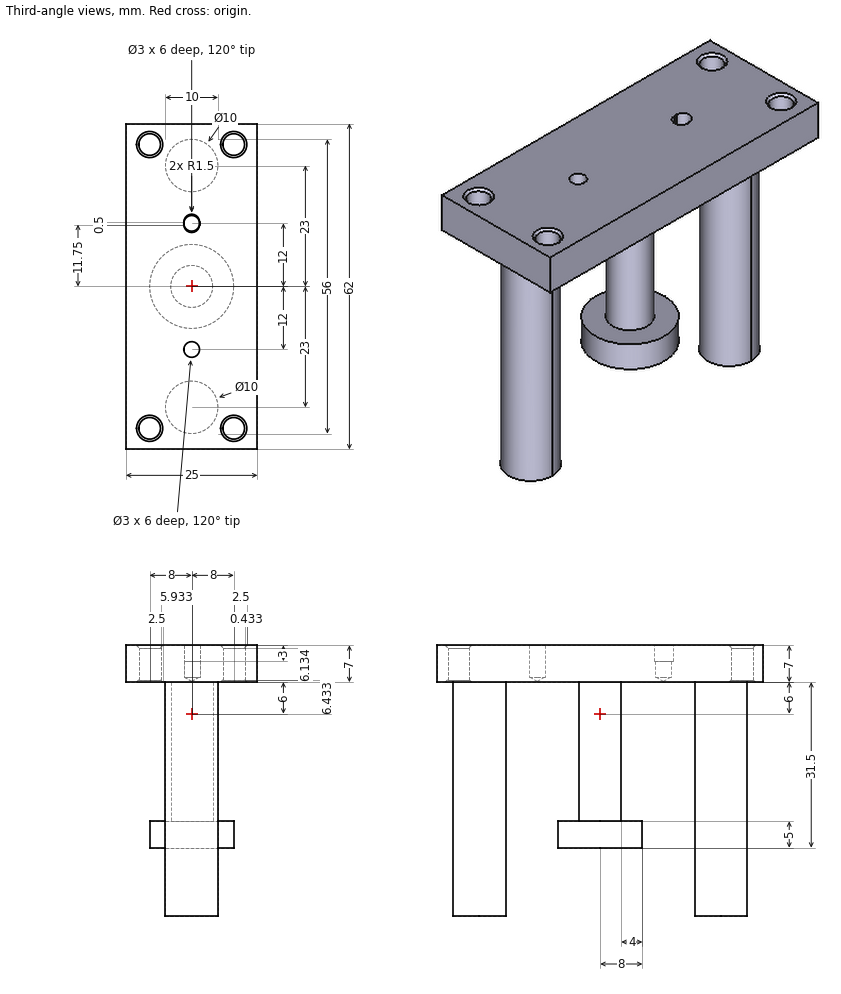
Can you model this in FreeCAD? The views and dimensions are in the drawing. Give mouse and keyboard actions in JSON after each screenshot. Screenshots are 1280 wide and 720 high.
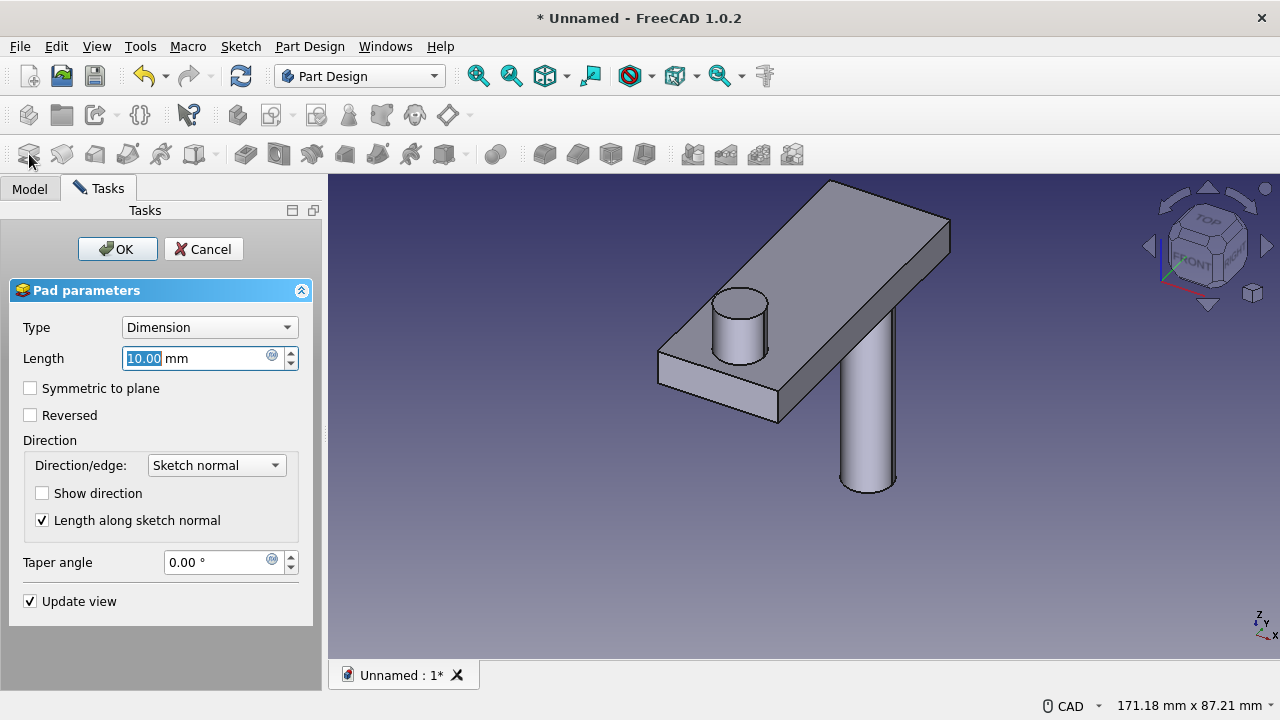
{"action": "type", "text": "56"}
{"action": "key", "text": "Tab"}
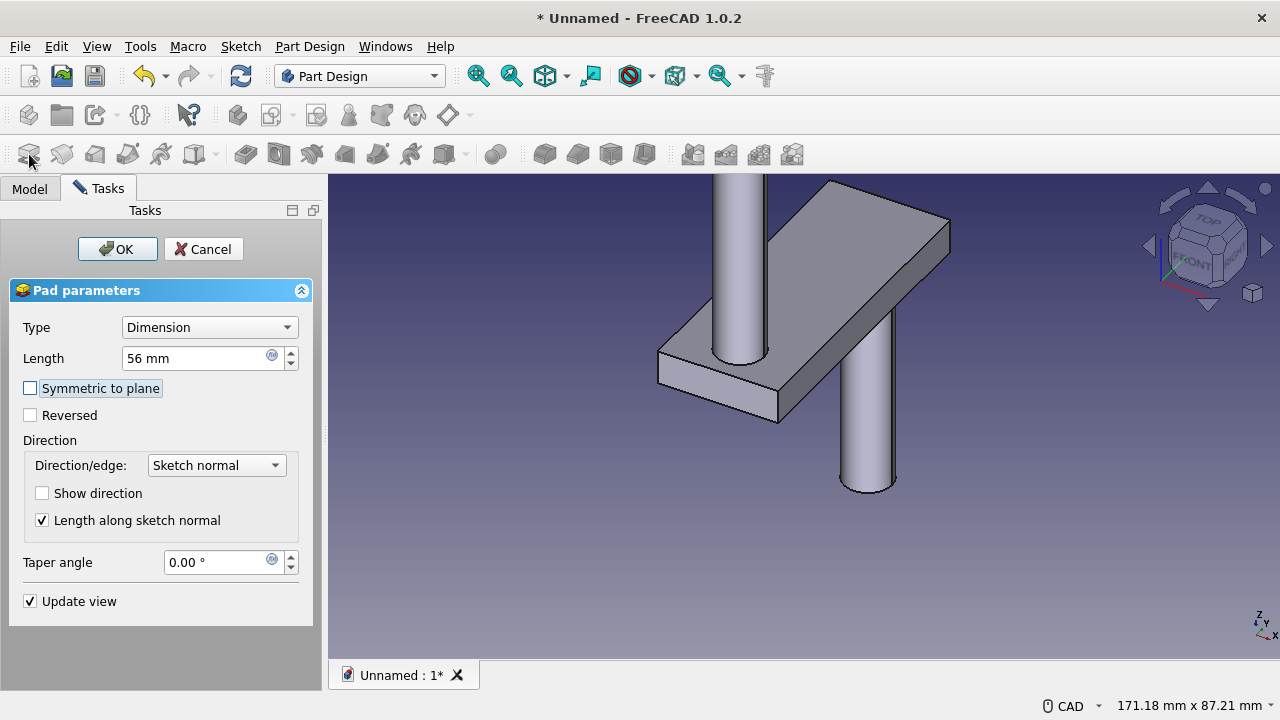
{"action": "left_click", "coordinate": [31, 415]}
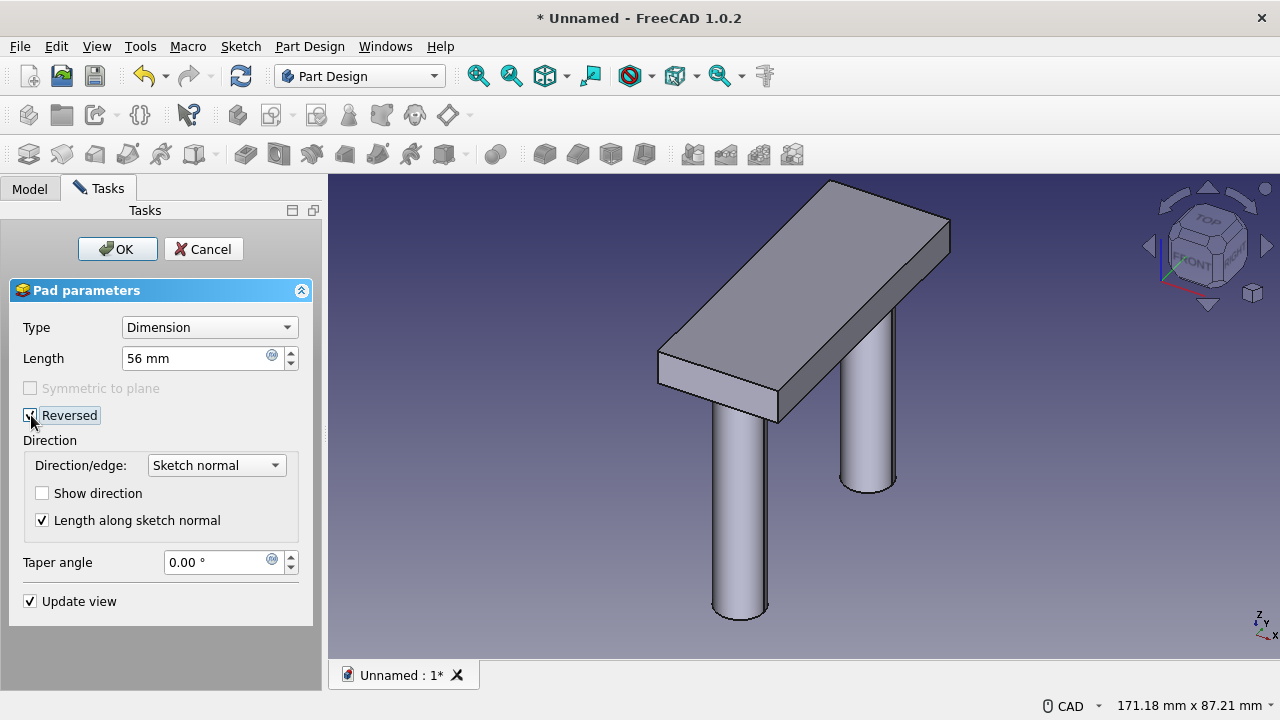
{"action": "left_click", "coordinate": [118, 249]}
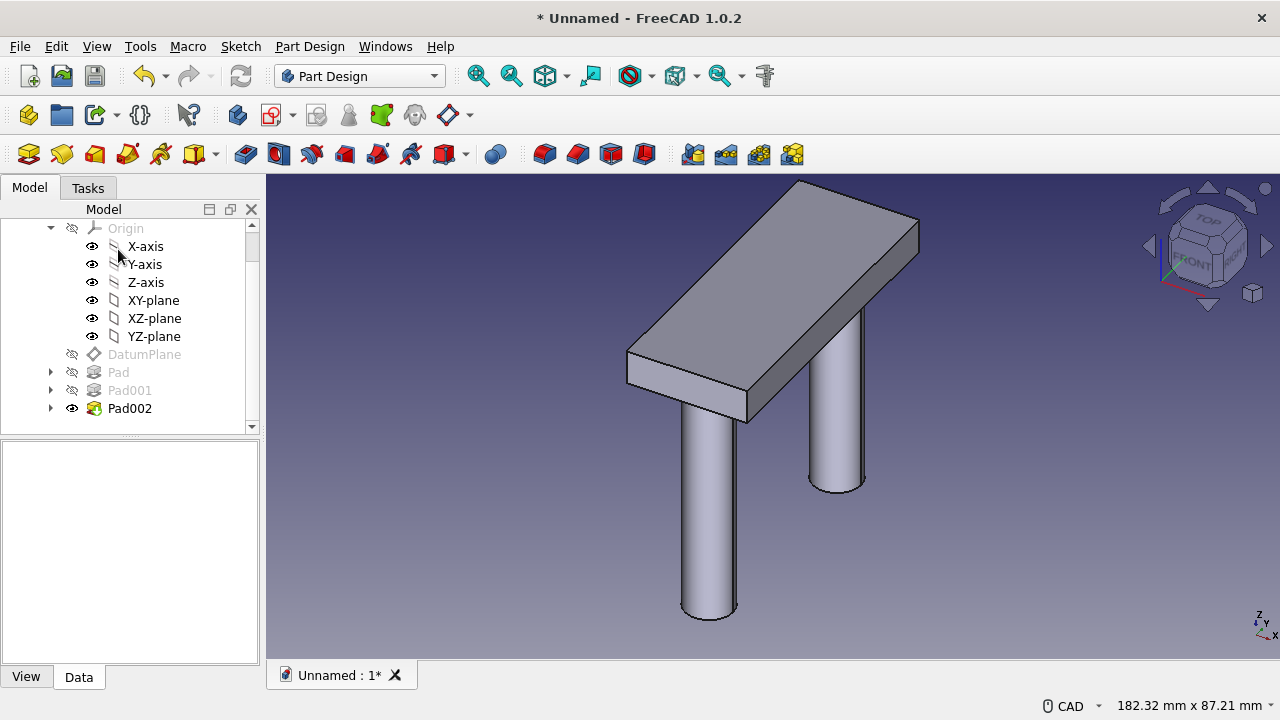
{"action": "left_click", "coordinate": [270, 116]}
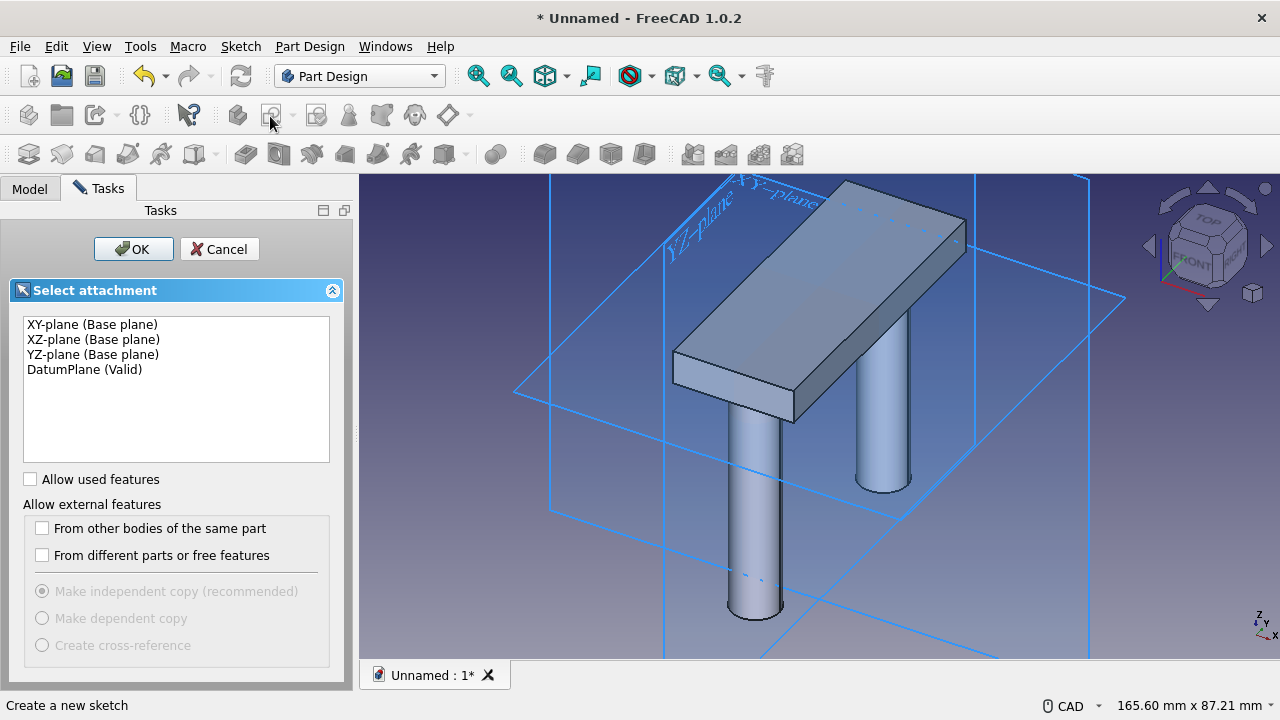
{"action": "left_click", "coordinate": [84, 354]}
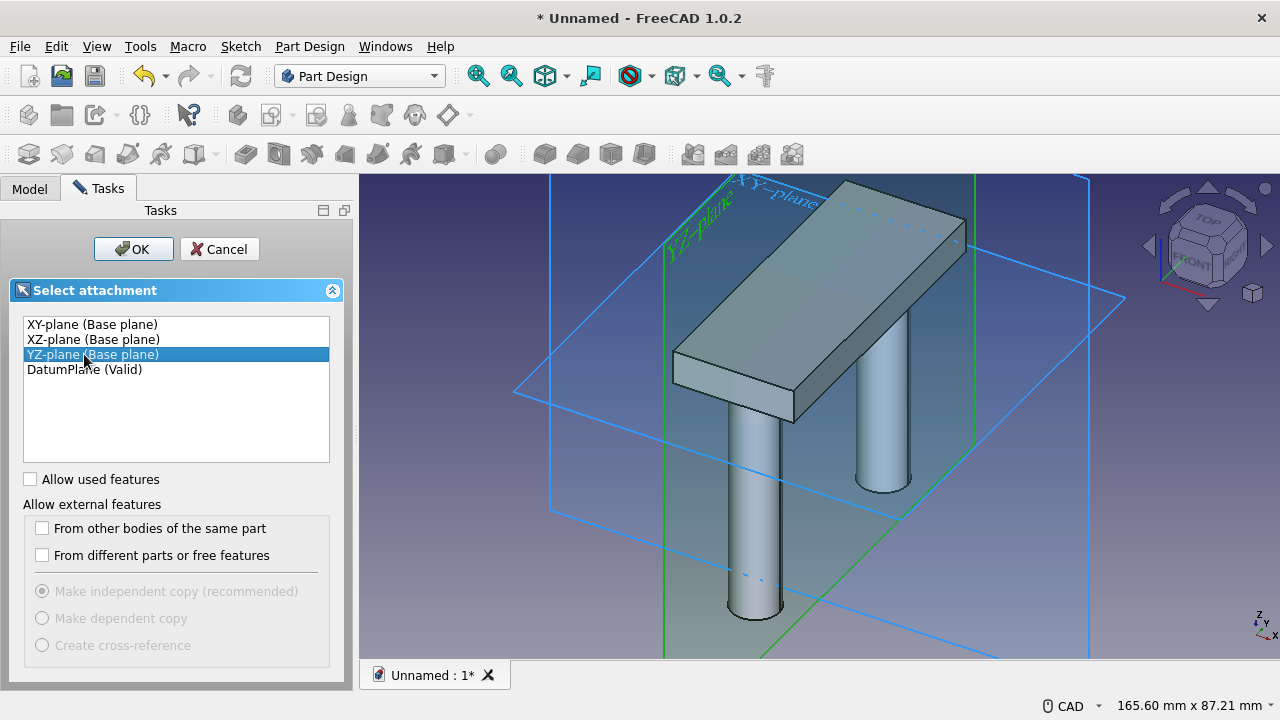
{"action": "left_click", "coordinate": [134, 249]}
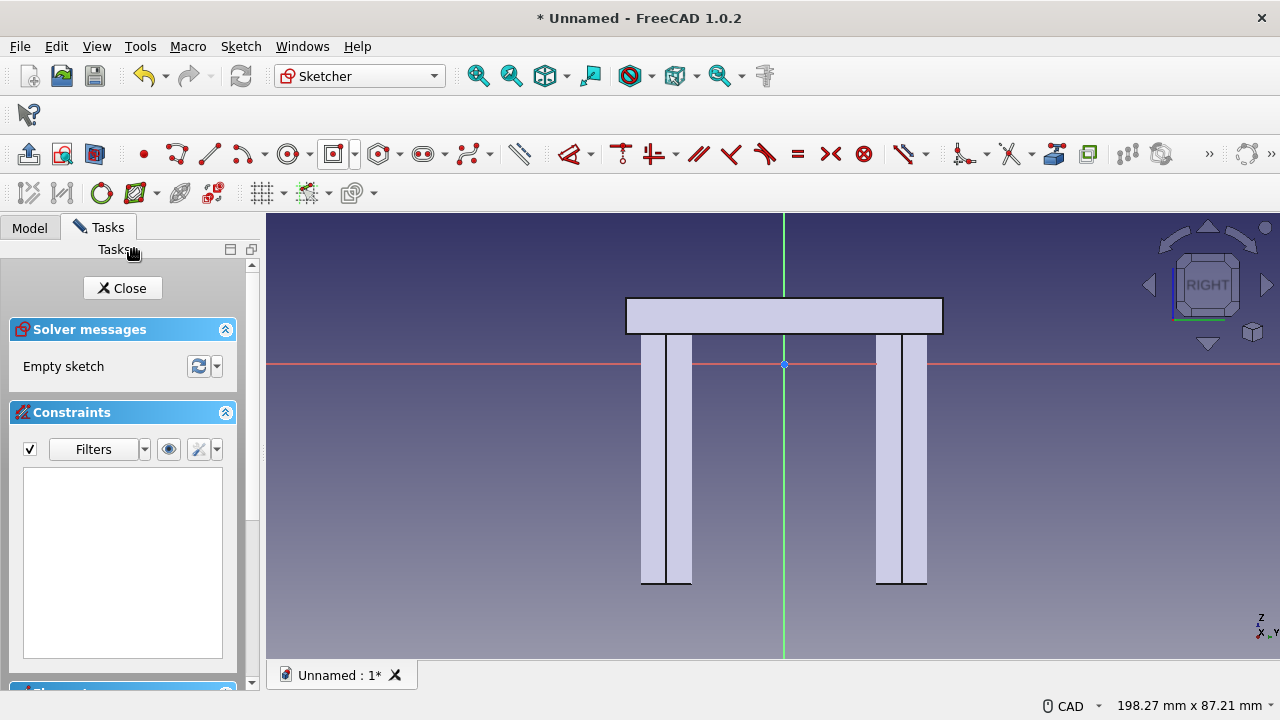
{"action": "left_click", "coordinate": [95, 154]}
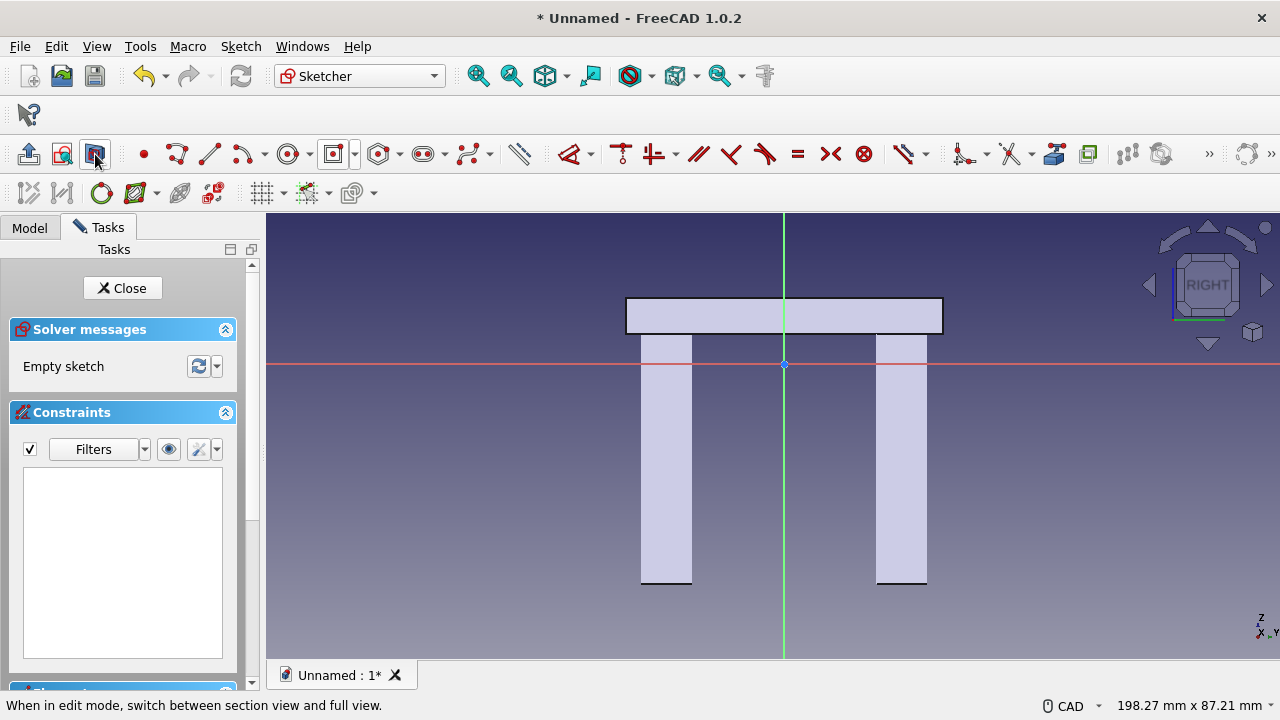
{"action": "scroll", "coordinate": [926, 388], "scroll_direction": "up", "scroll_amount": 3}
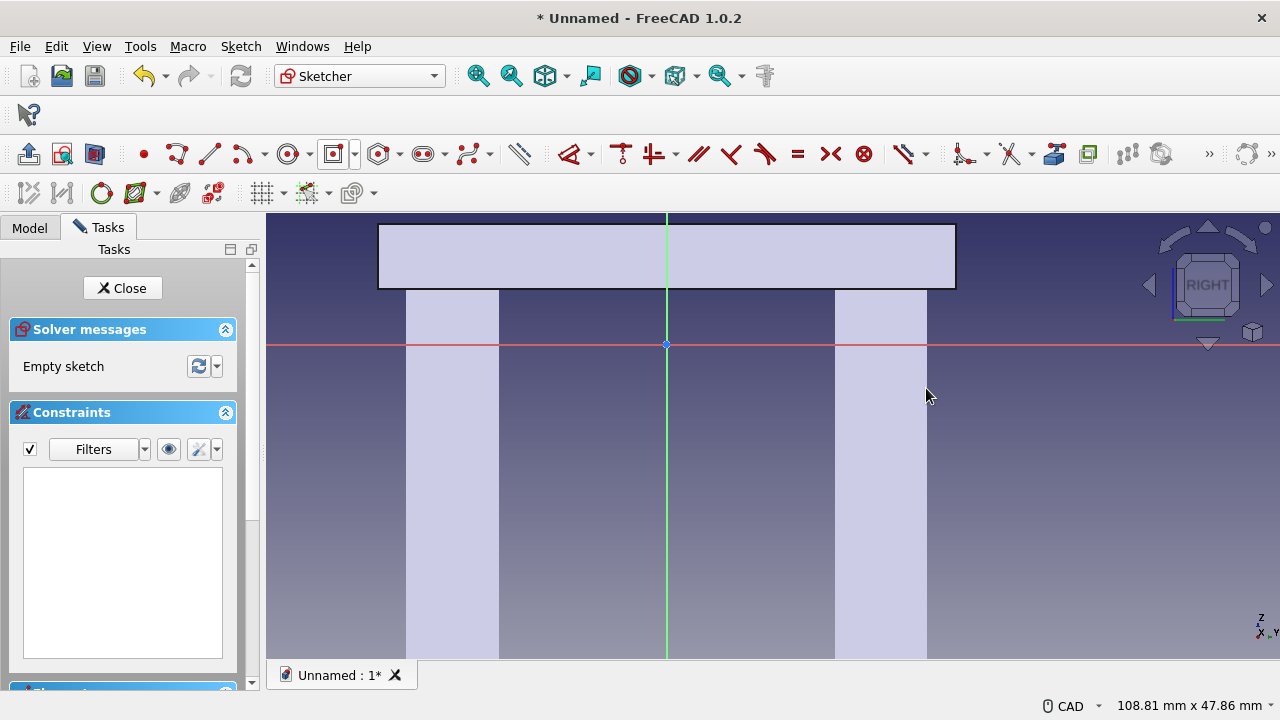
{"action": "left_click", "coordinate": [177, 154]}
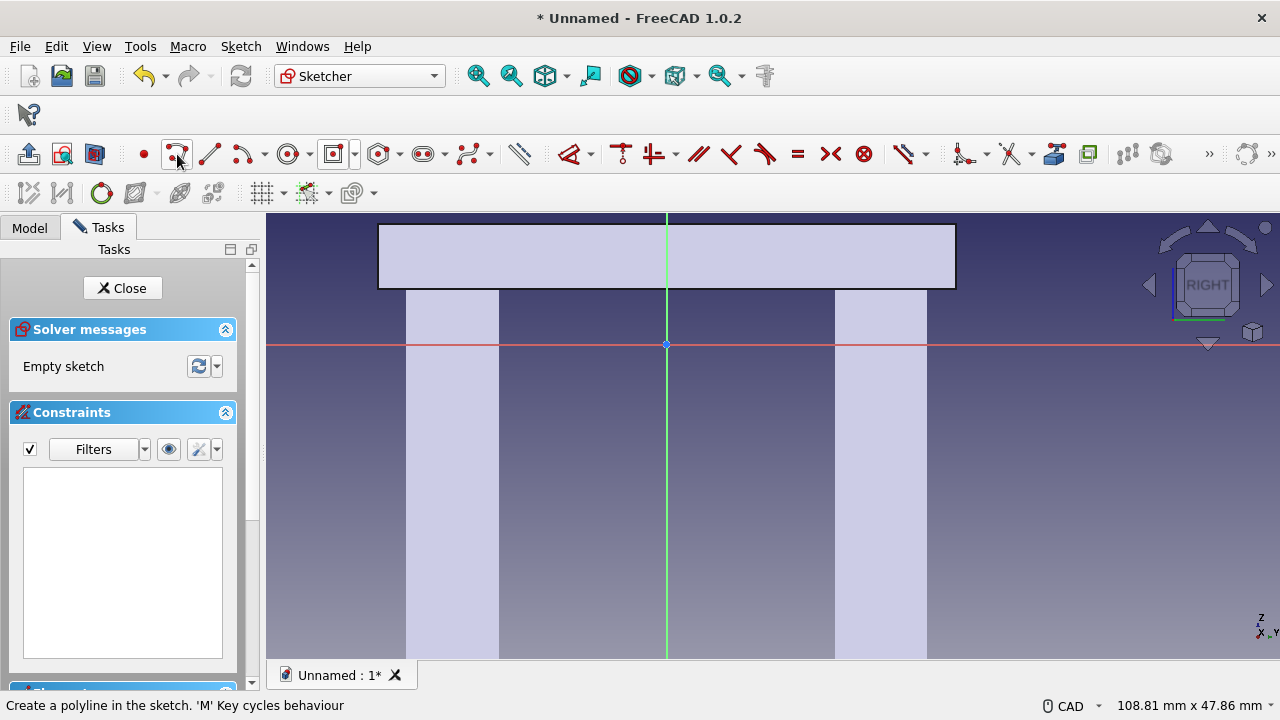
{"action": "left_click", "coordinate": [667, 289]}
{"action": "left_click", "coordinate": [676, 582]}
{"action": "left_click", "coordinate": [741, 582]}
{"action": "left_click", "coordinate": [741, 536]}
{"action": "left_click", "coordinate": [704, 536]}
{"action": "left_click", "coordinate": [704, 289]}
{"action": "left_click", "coordinate": [667, 290]}
{"action": "key", "text": "Escape"}
{"action": "key", "text": "Escape"}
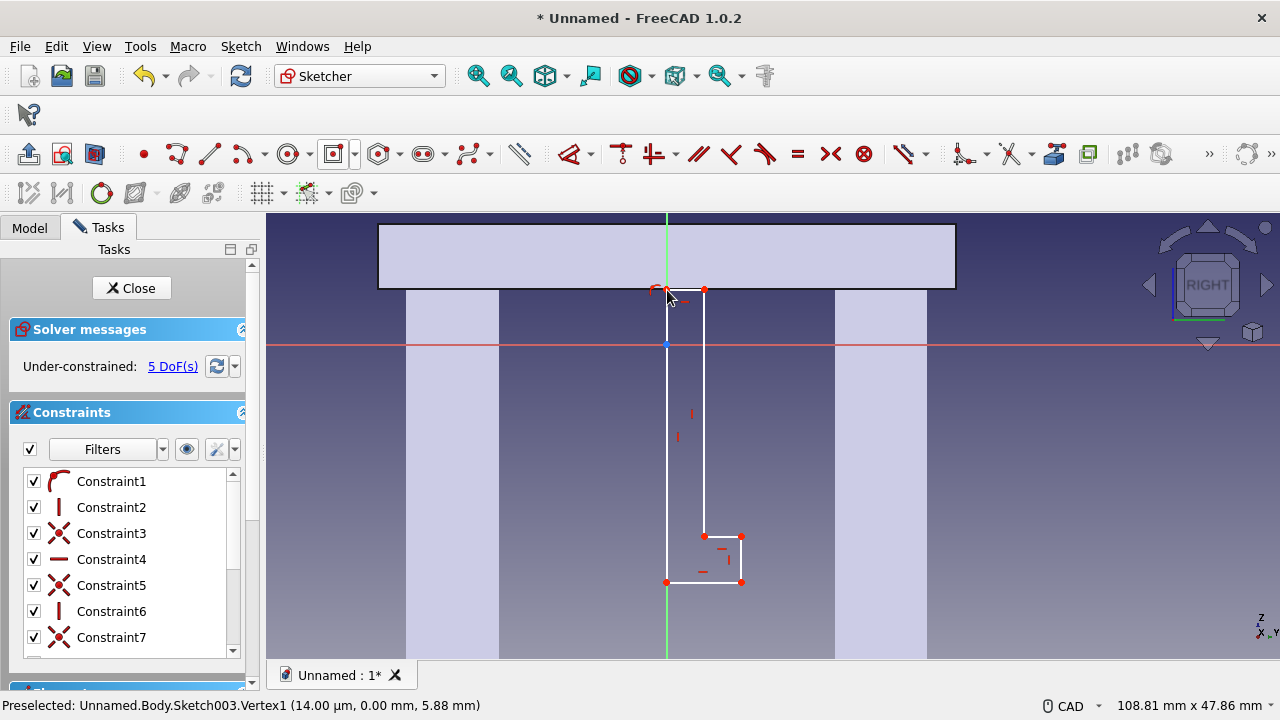
{"action": "left_click", "coordinate": [568, 154]}